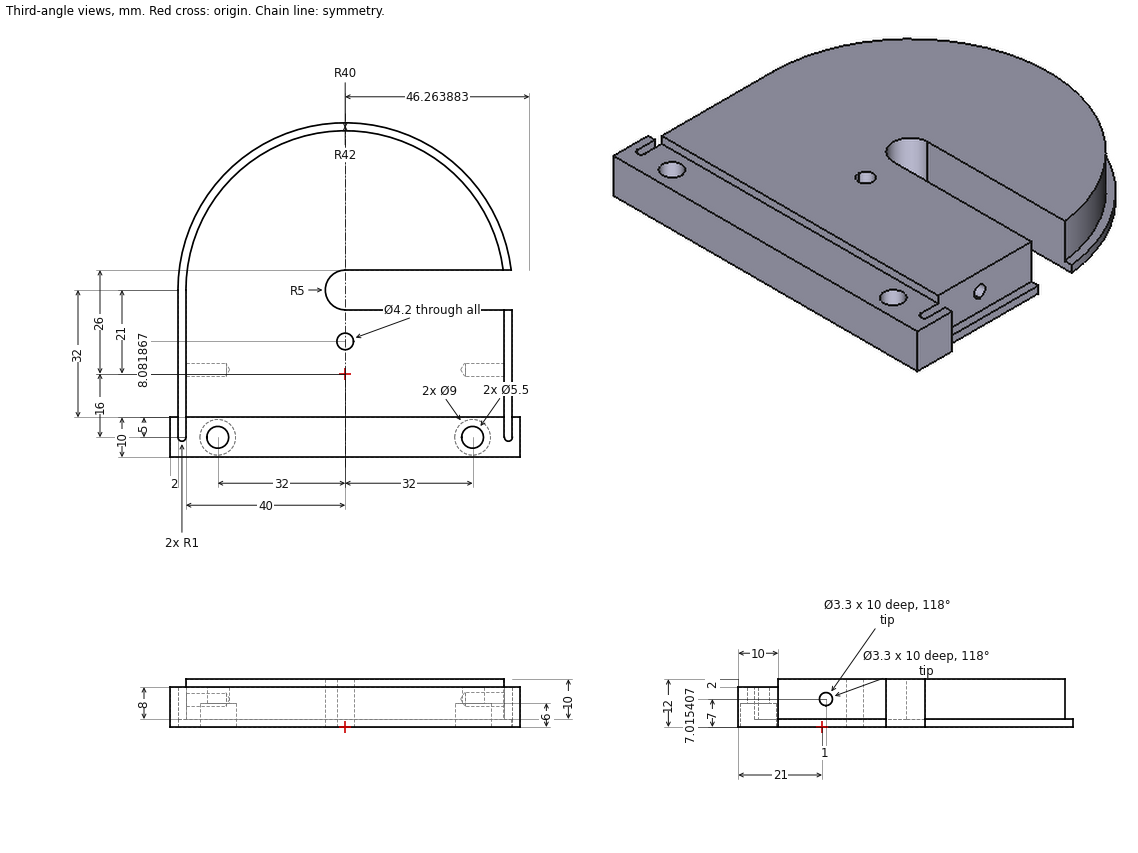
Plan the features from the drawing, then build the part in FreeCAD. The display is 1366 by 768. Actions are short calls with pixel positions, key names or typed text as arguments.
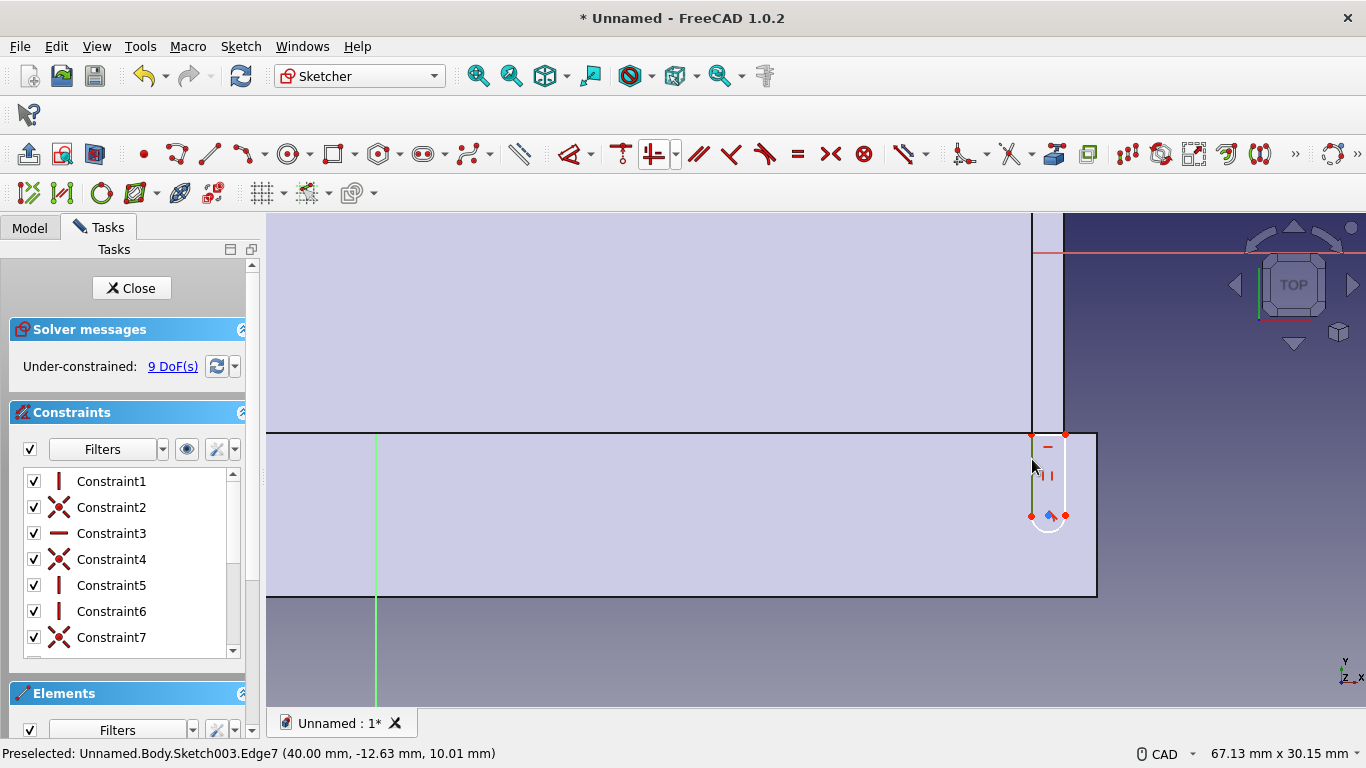
click(1039, 530)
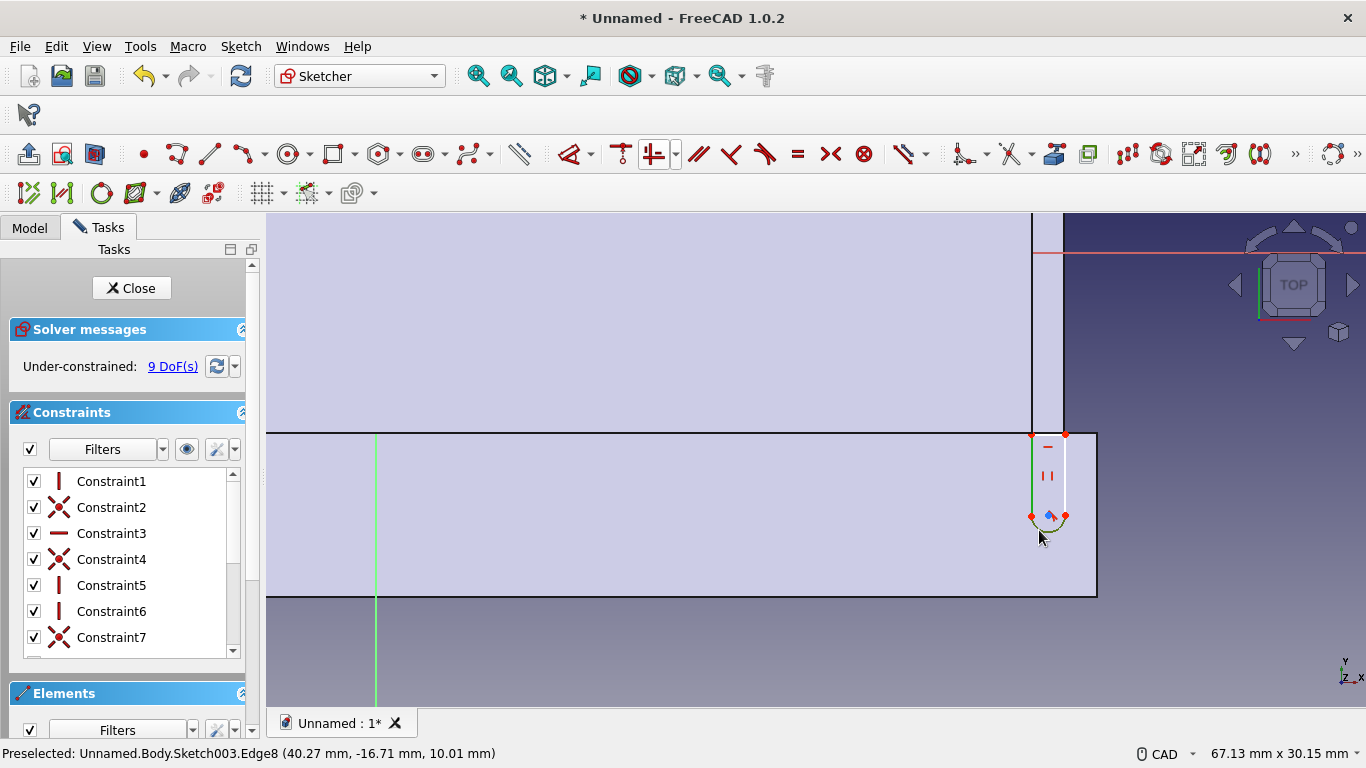
click(765, 154)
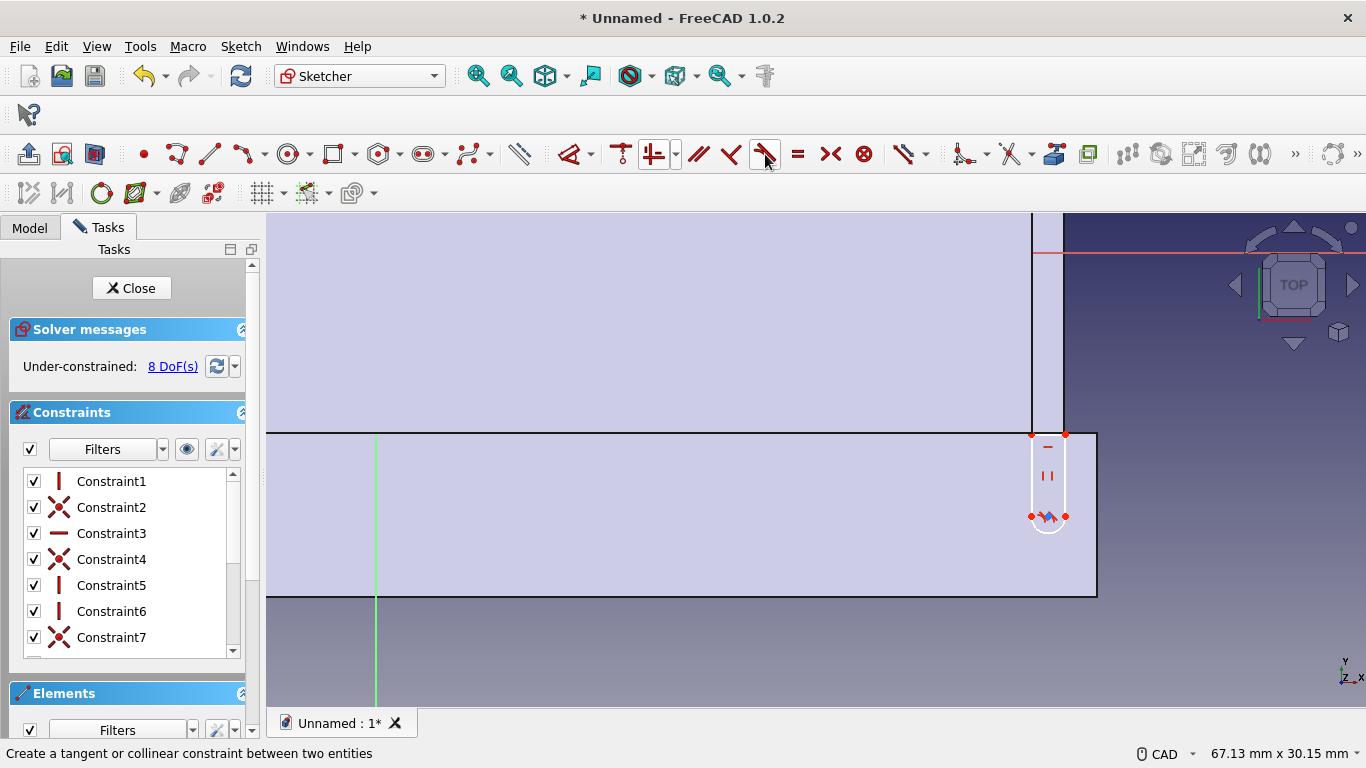
scroll(1051, 515, down, 4)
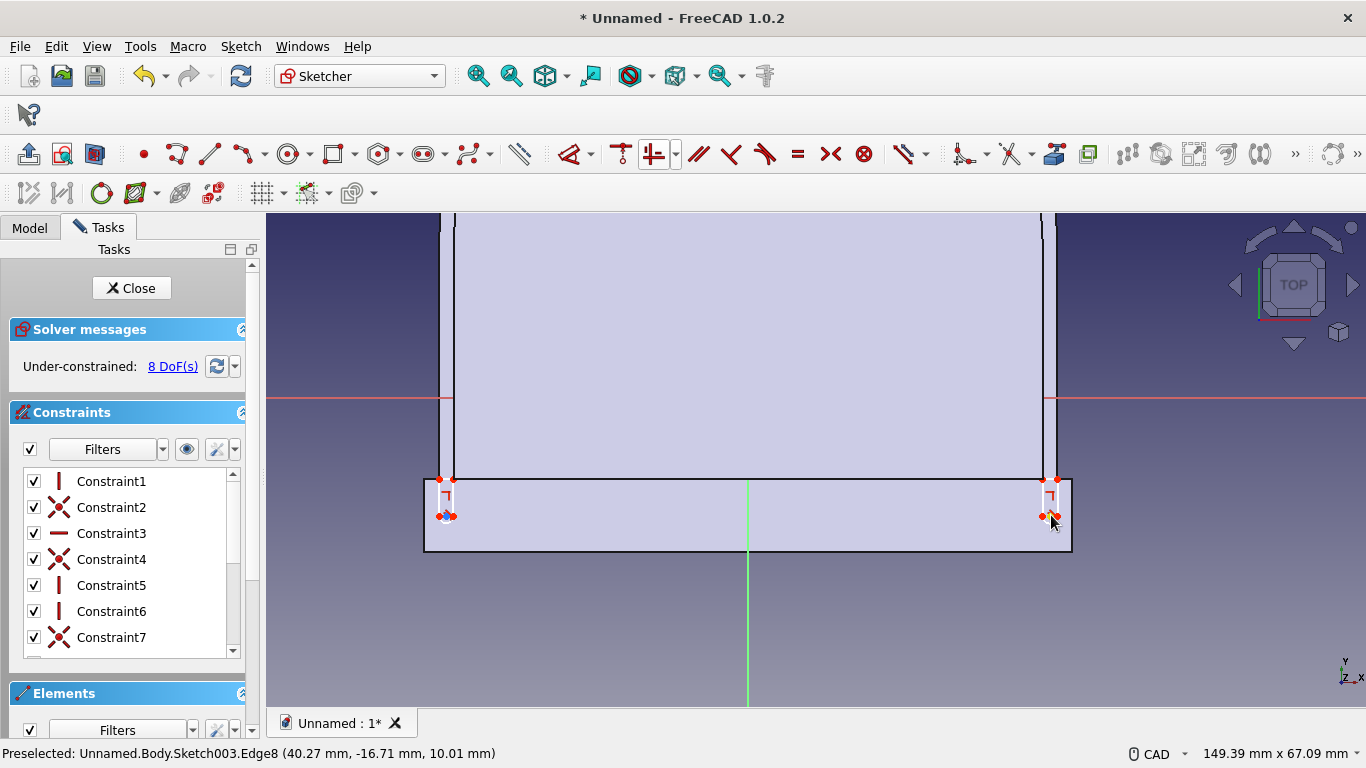
scroll(442, 522, up, 4)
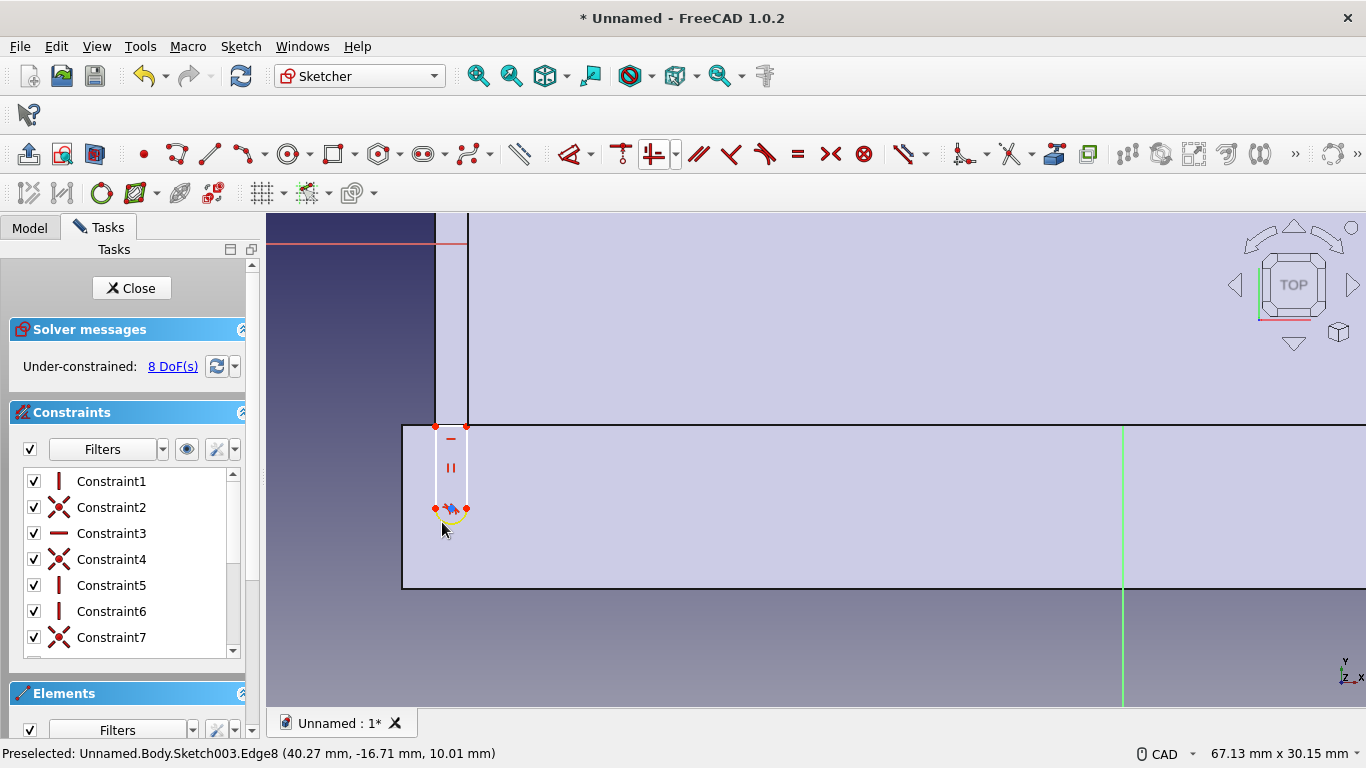
click(442, 521)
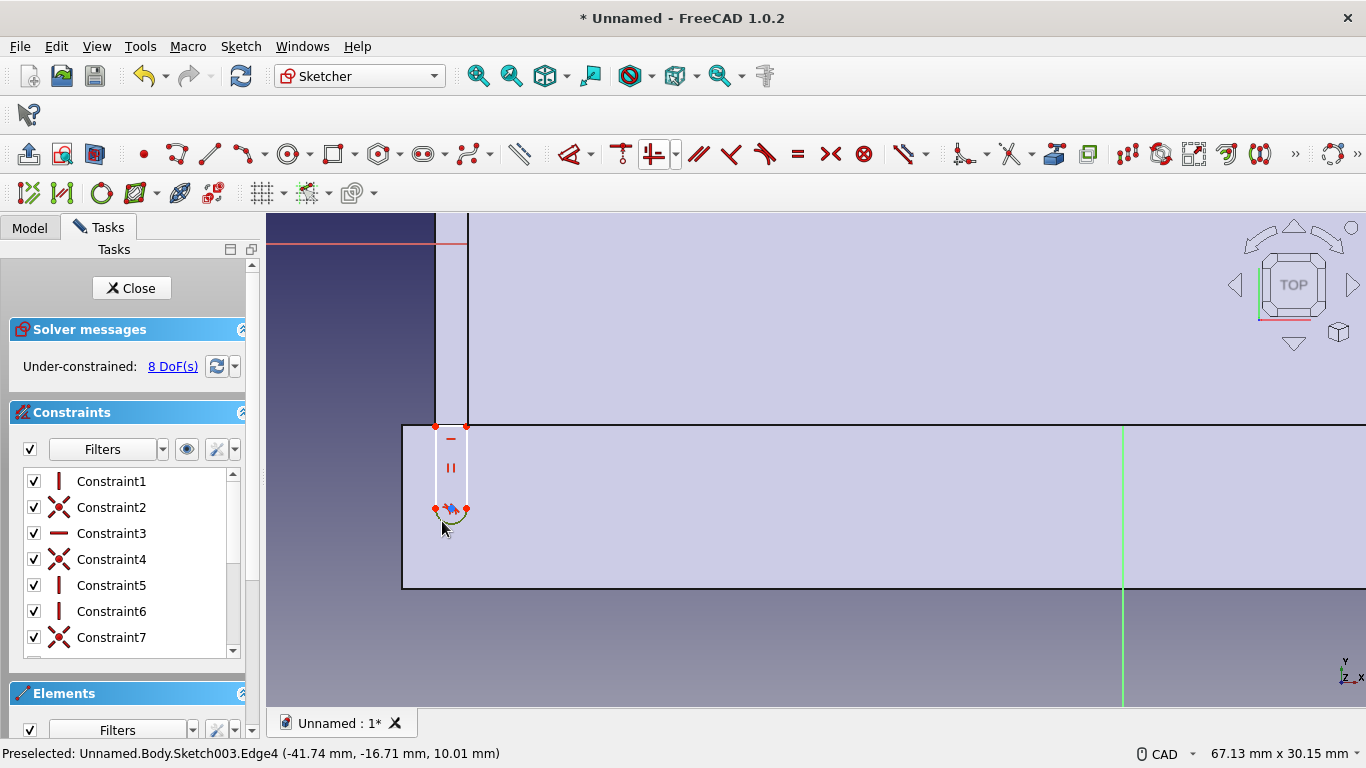
scroll(441, 522, down, 4)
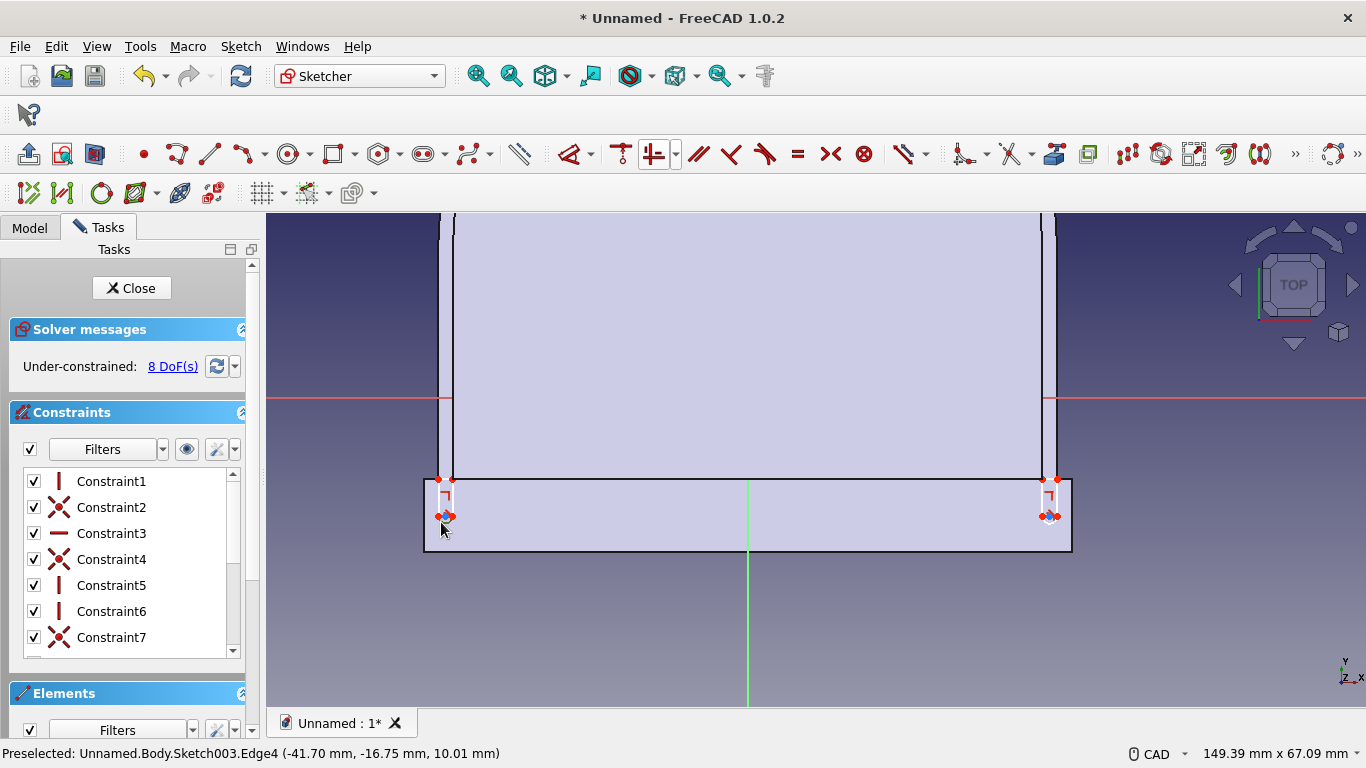
scroll(1045, 522, up, 4)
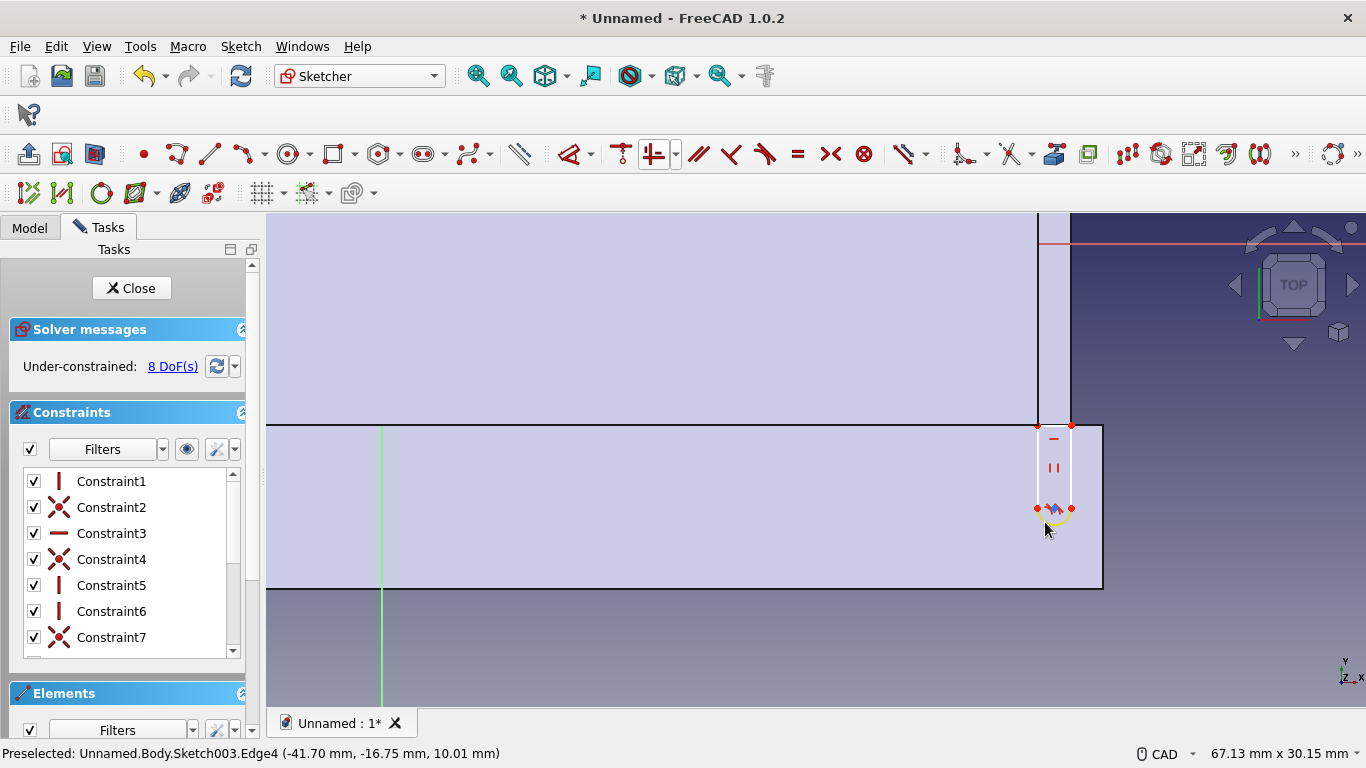
click(1045, 522)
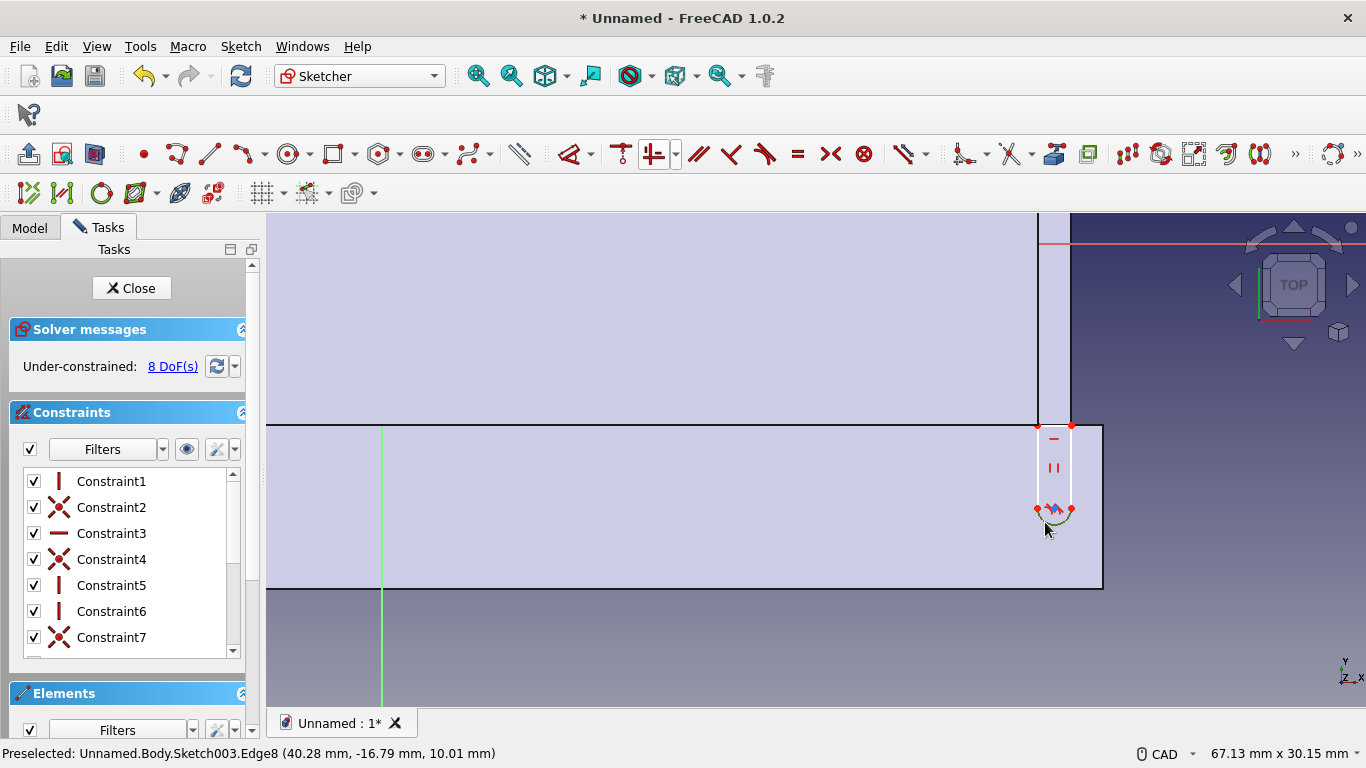
click(798, 154)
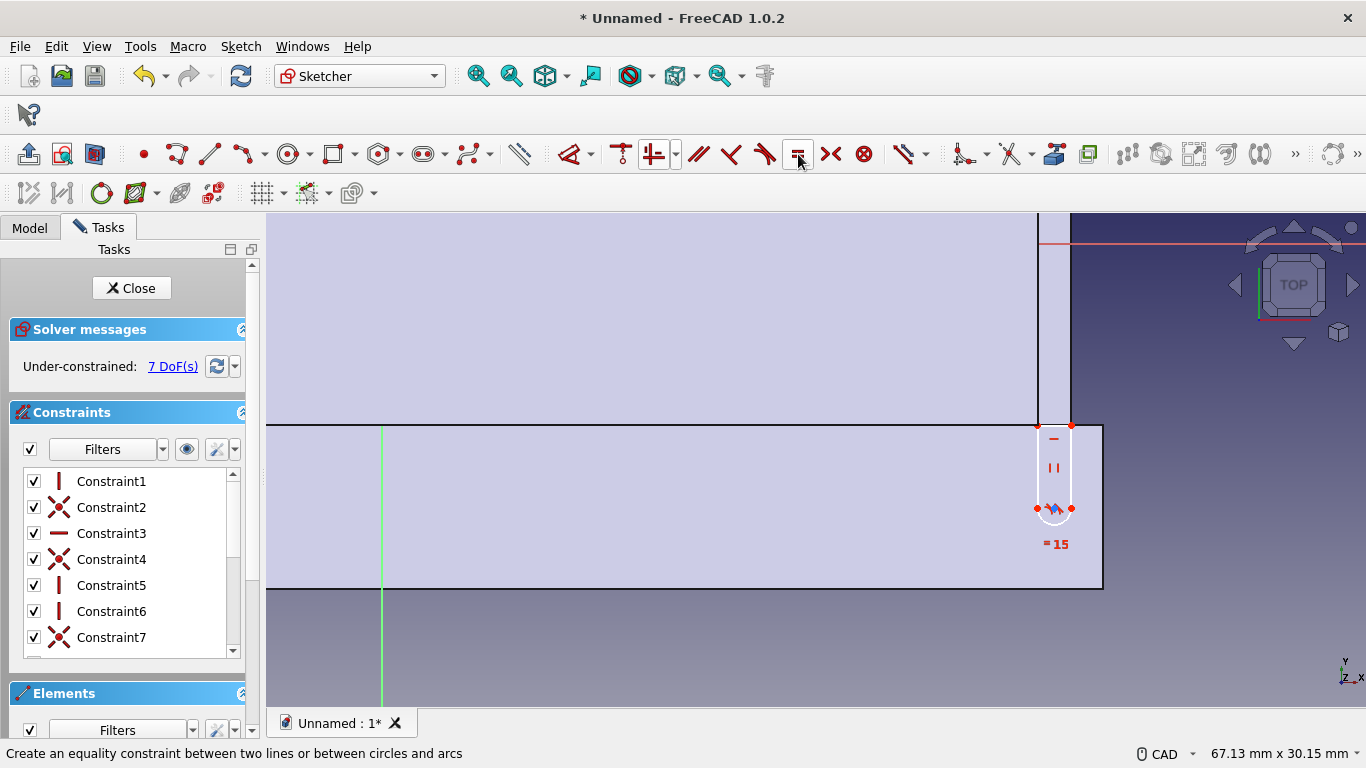
scroll(1046, 522, down, 4)